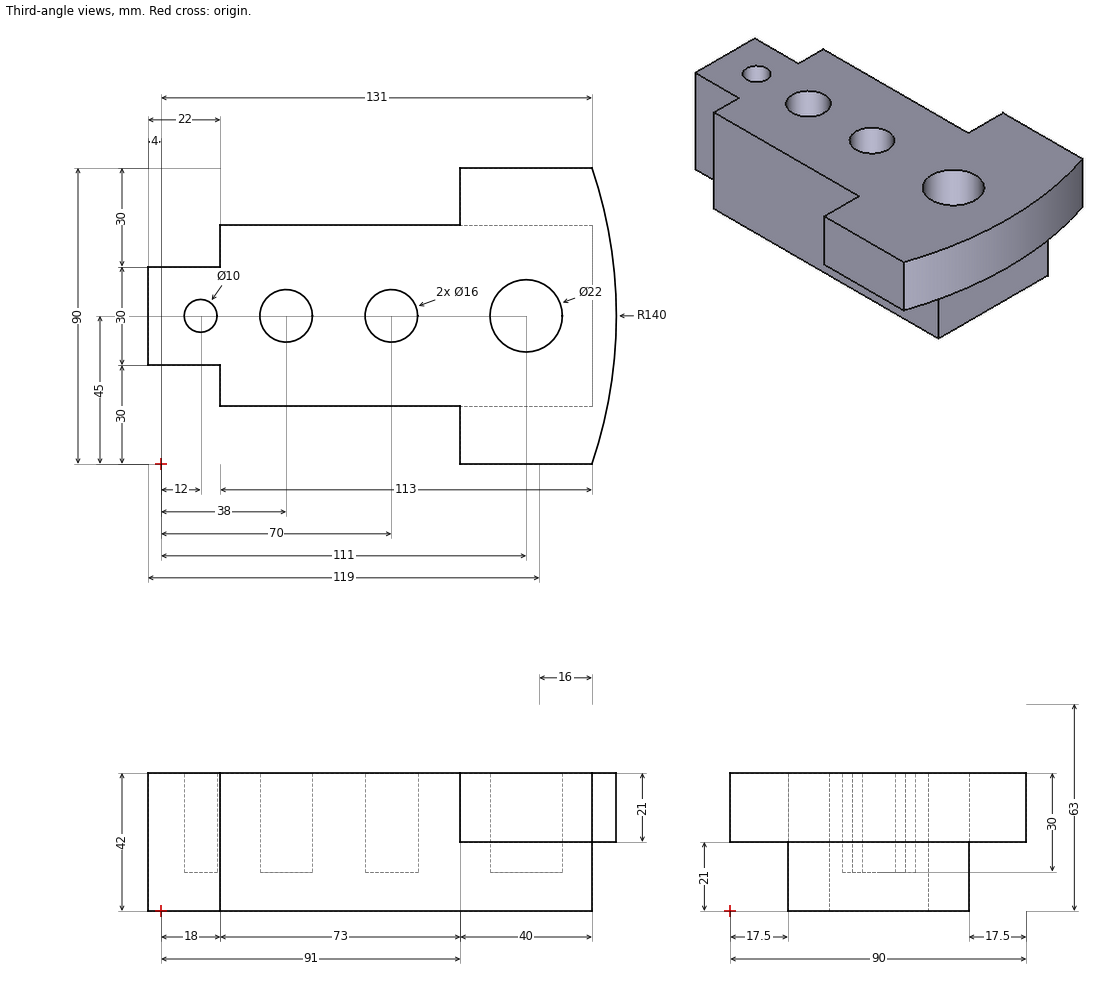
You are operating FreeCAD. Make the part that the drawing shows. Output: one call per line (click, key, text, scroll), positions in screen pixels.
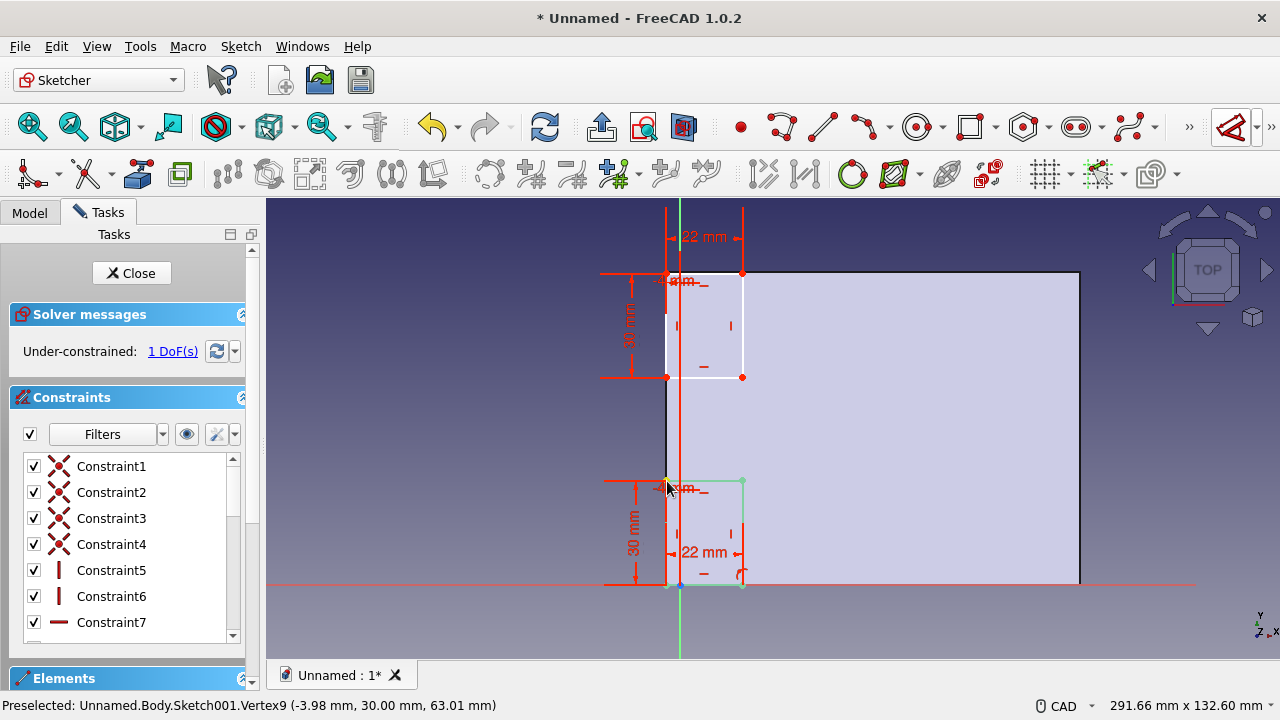
click(666, 274)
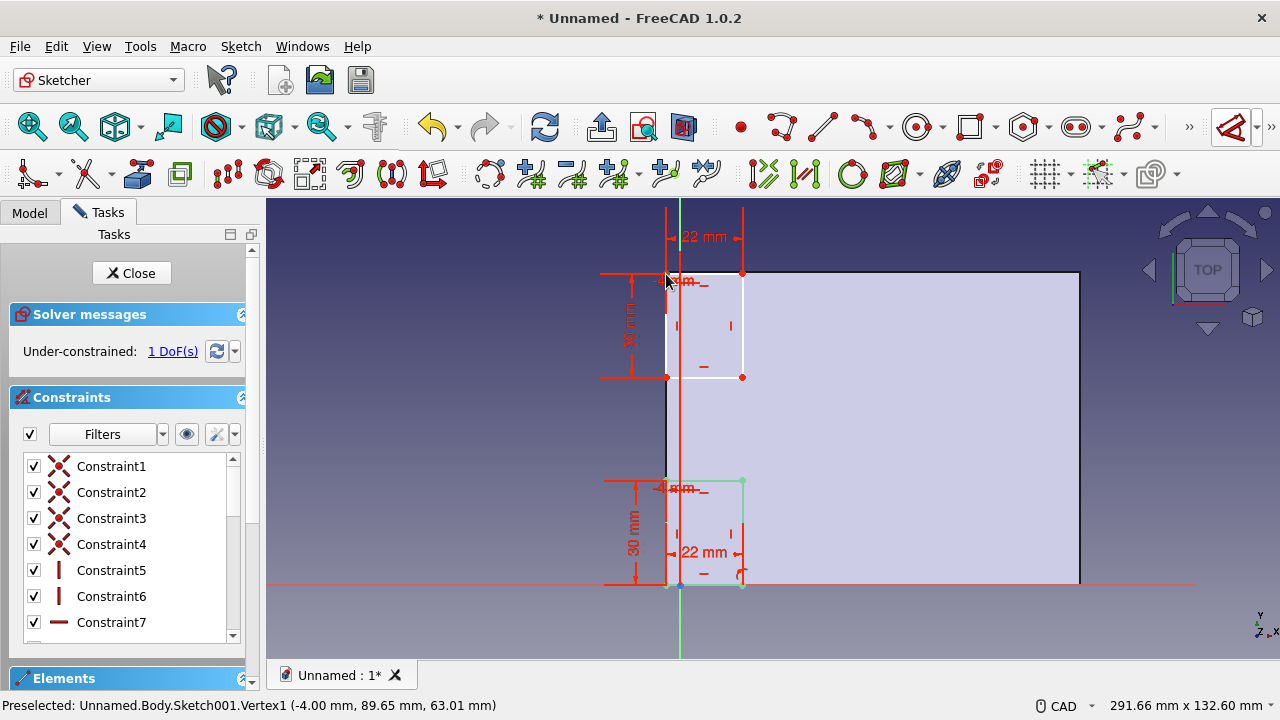
key(i)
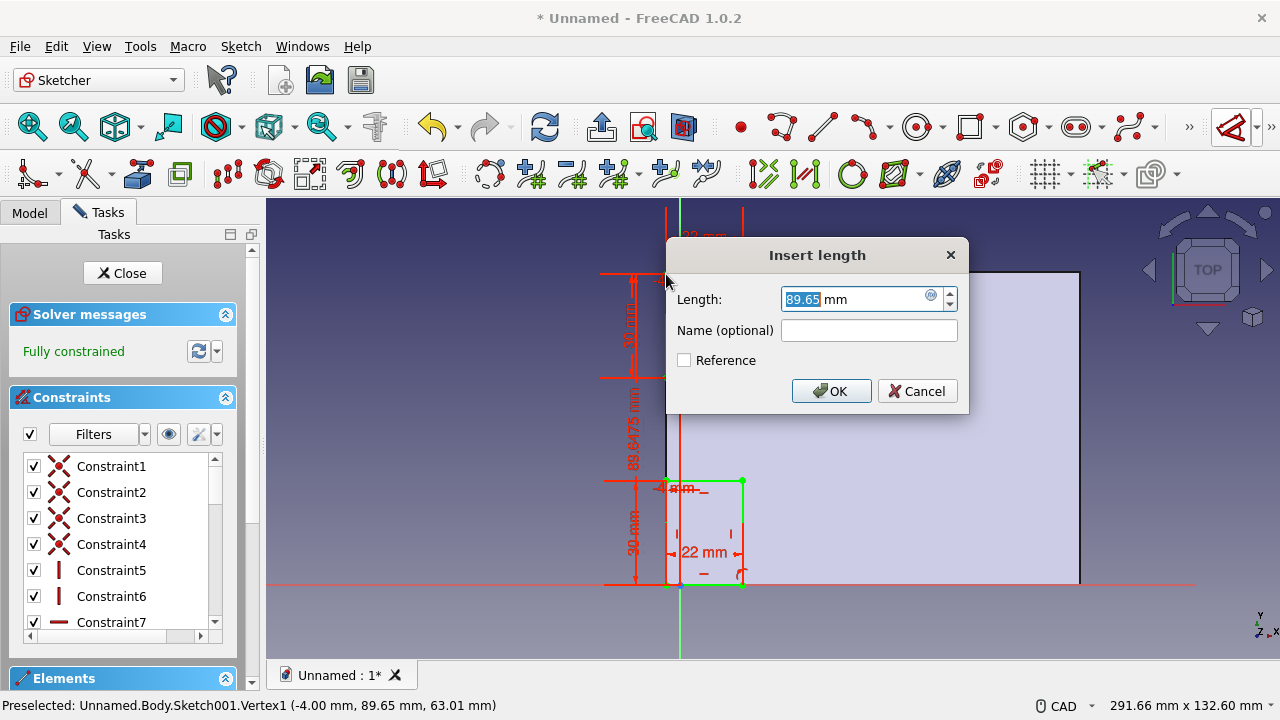
text(90)
key(Return)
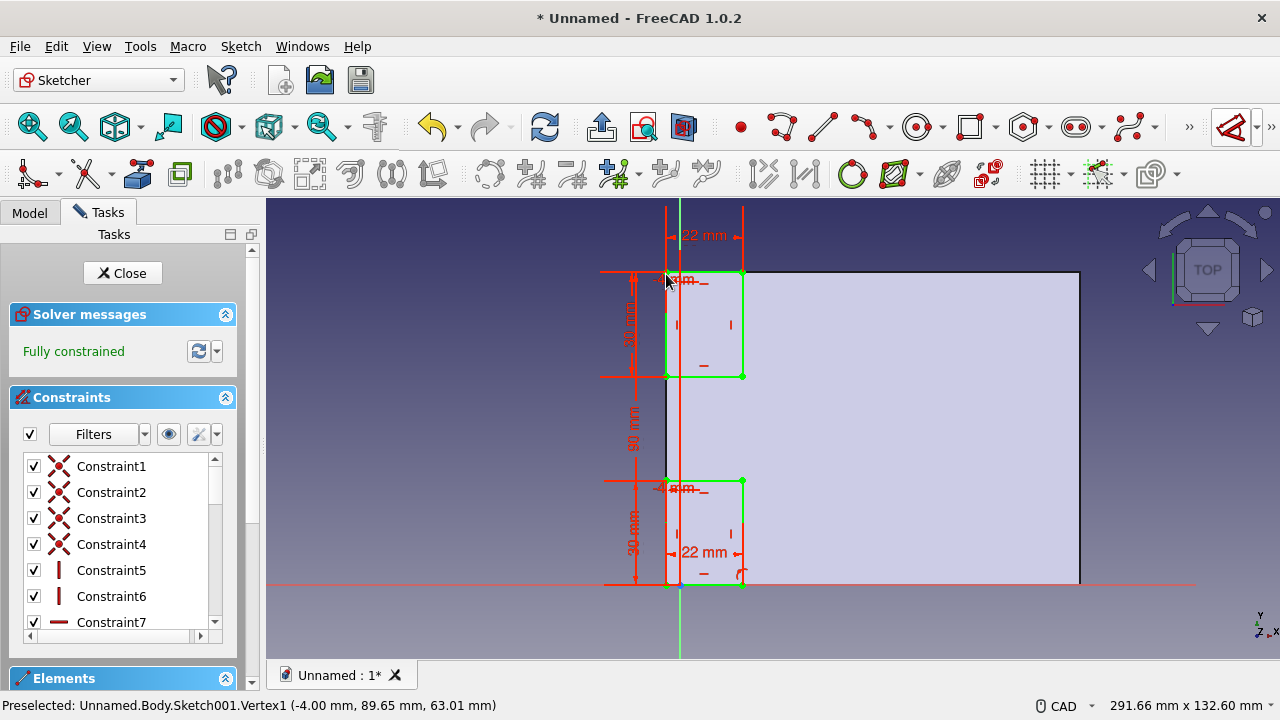
click(123, 273)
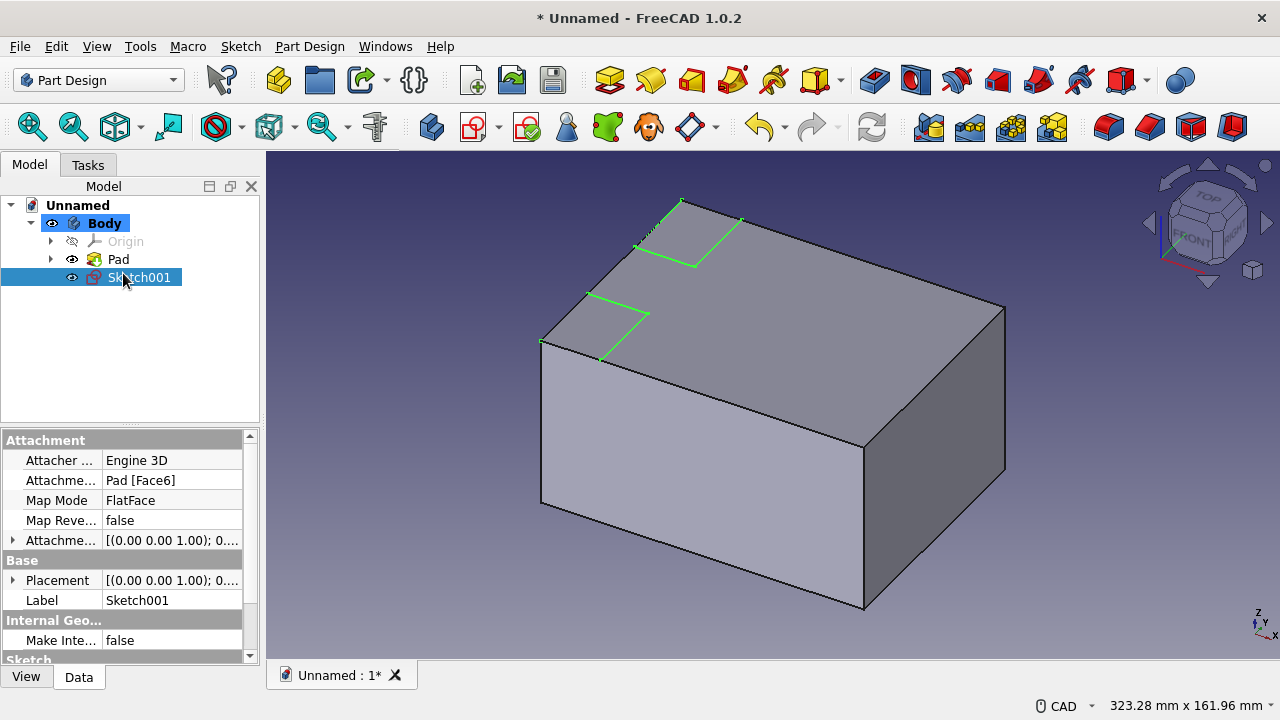
click(875, 80)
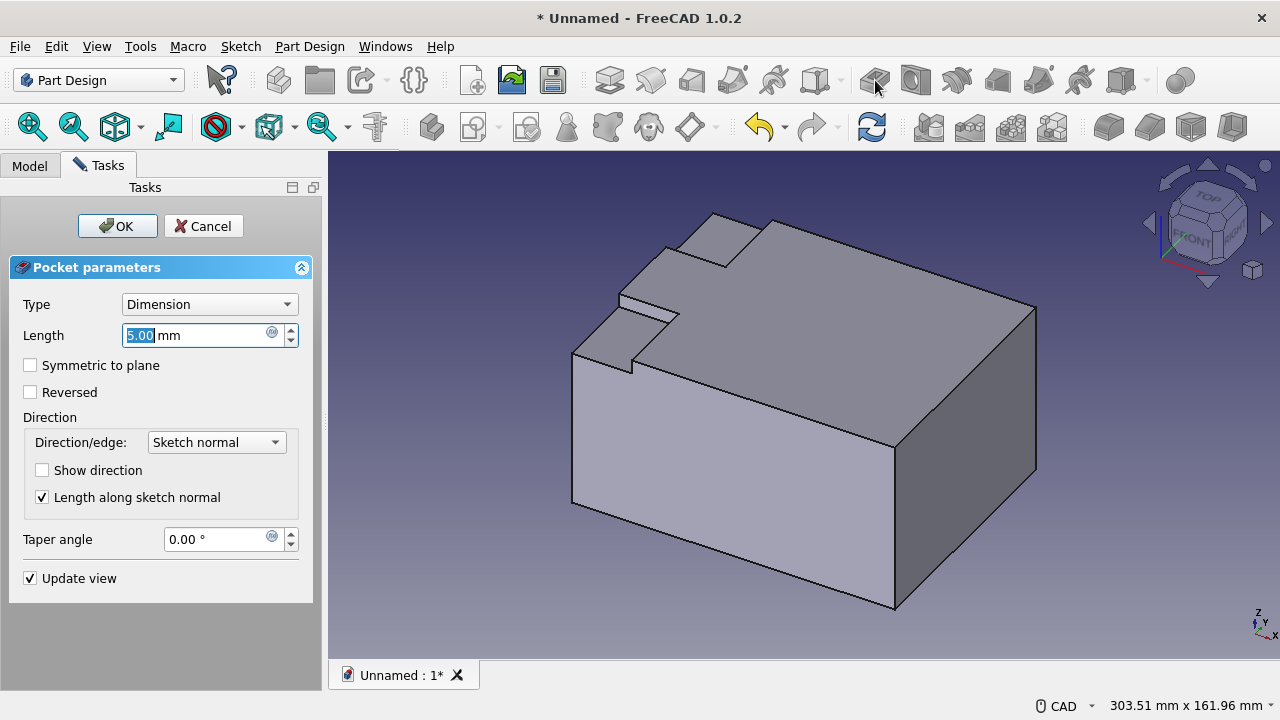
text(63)
key(Tab)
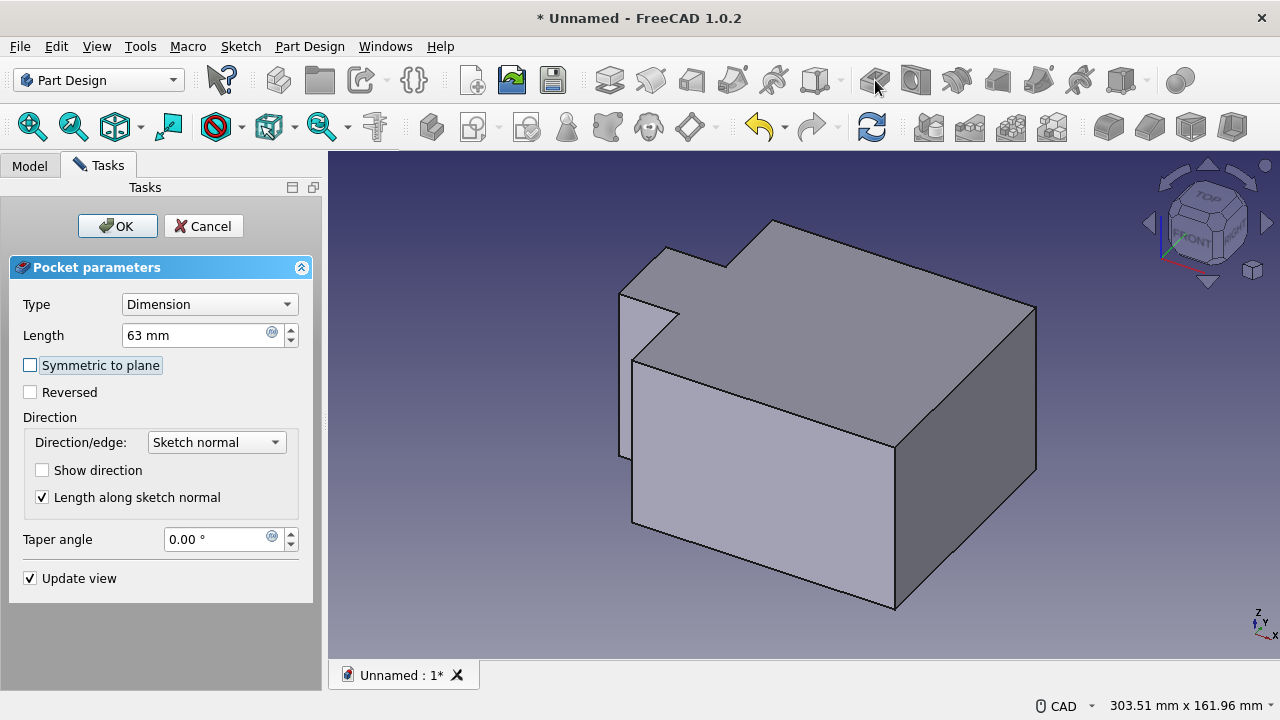
click(118, 226)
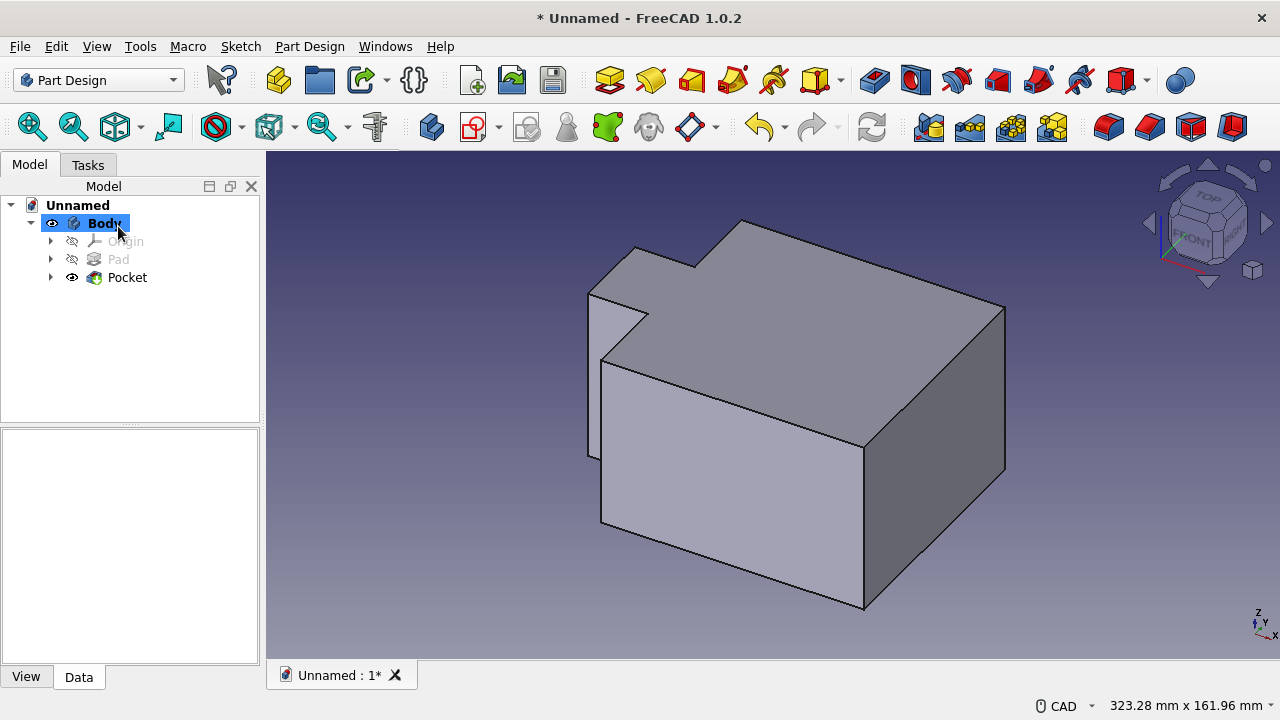
click(955, 437)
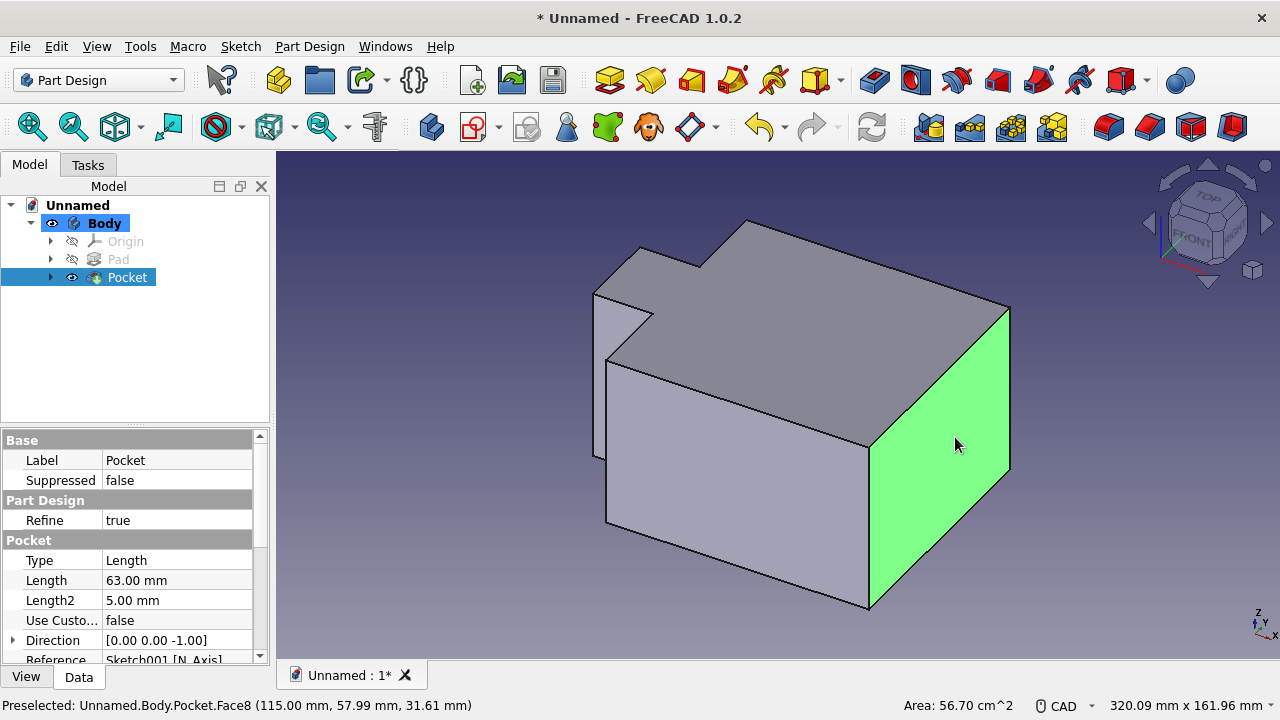
click(472, 128)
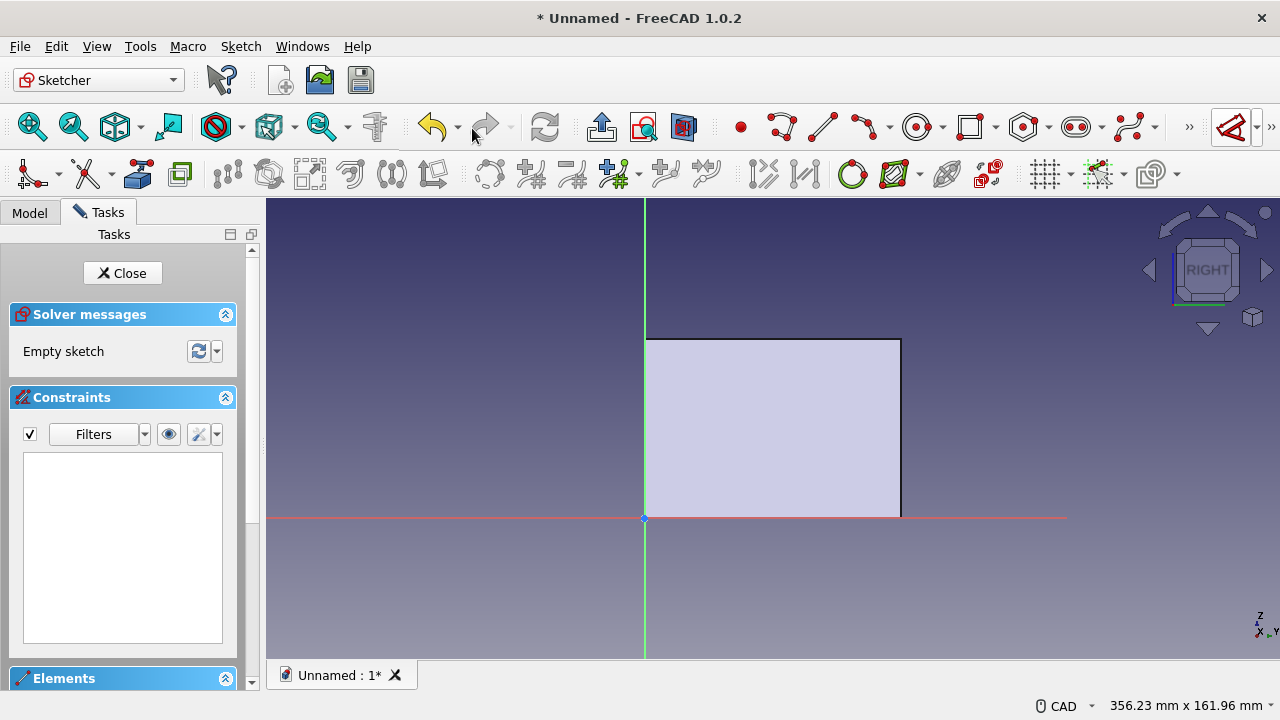
scroll(912, 428, up, 2)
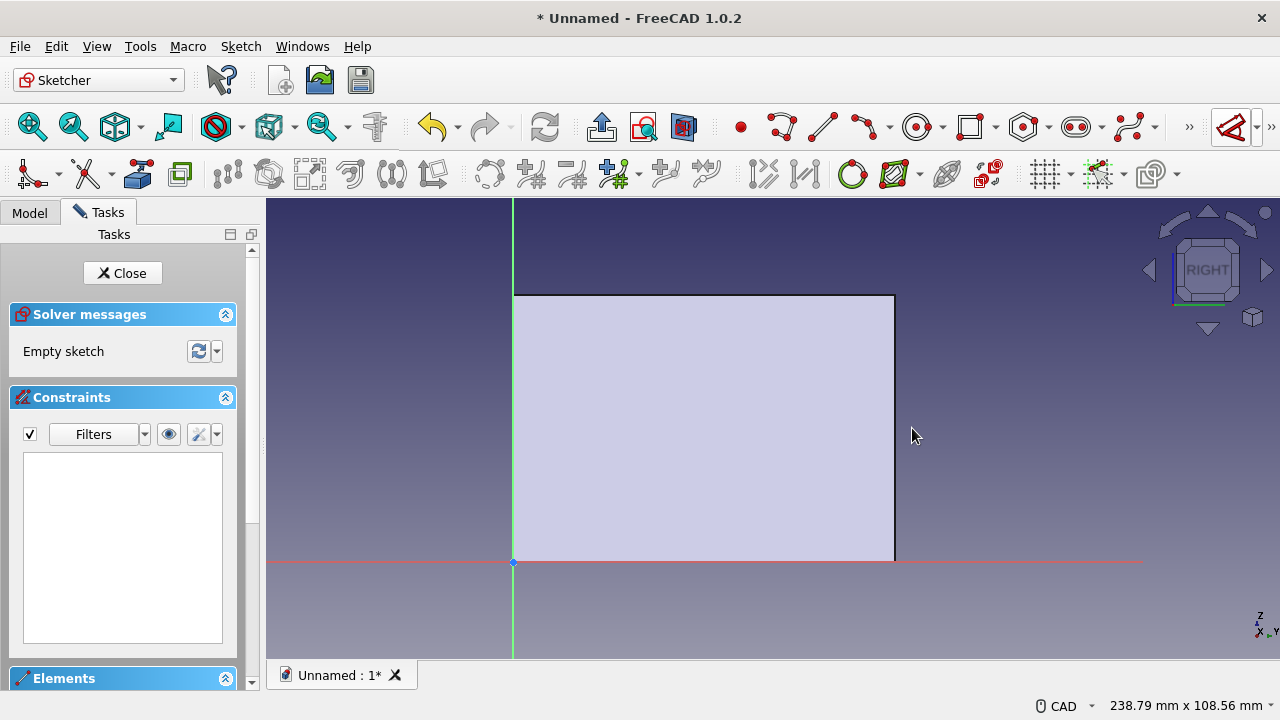
click(970, 128)